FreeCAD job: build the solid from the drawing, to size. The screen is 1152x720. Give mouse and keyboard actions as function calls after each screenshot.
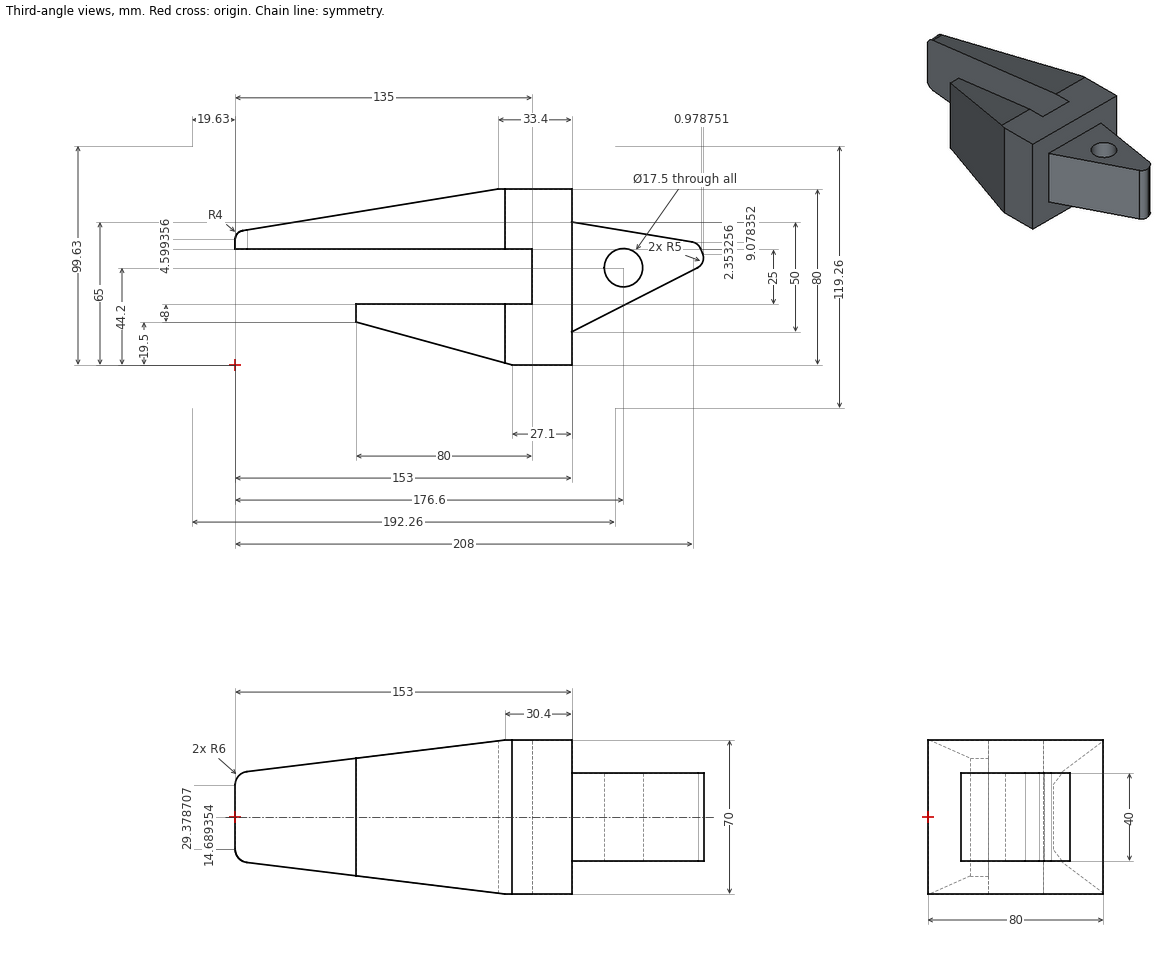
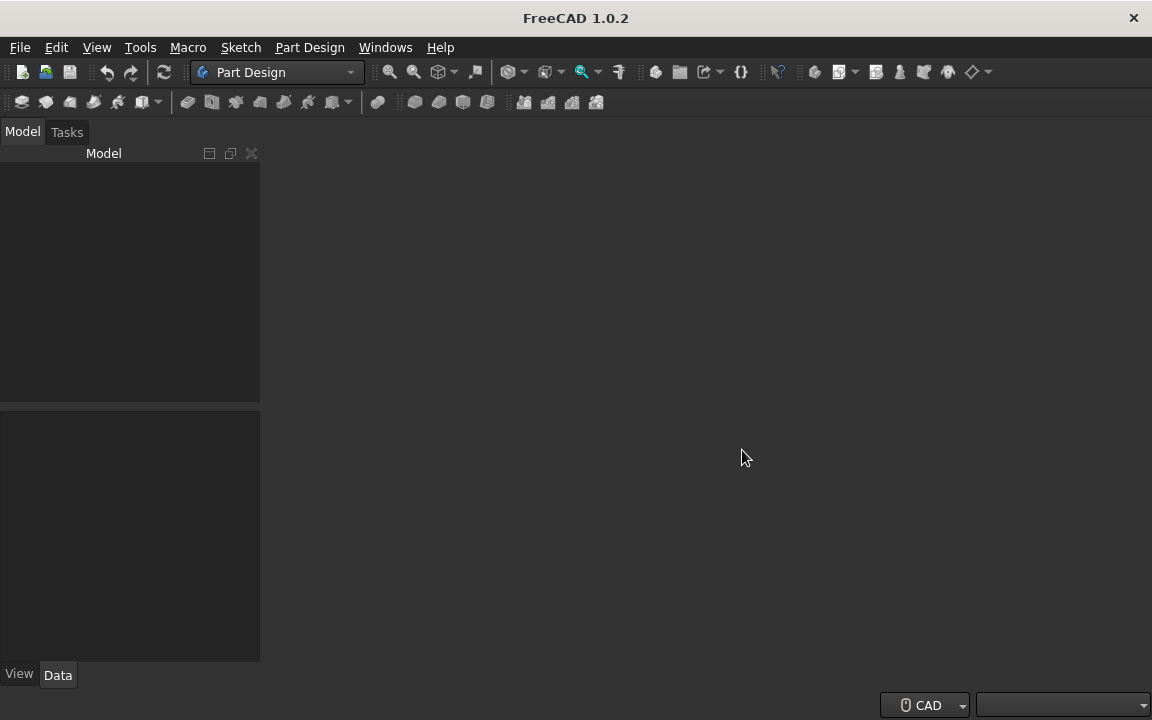
click(22, 72)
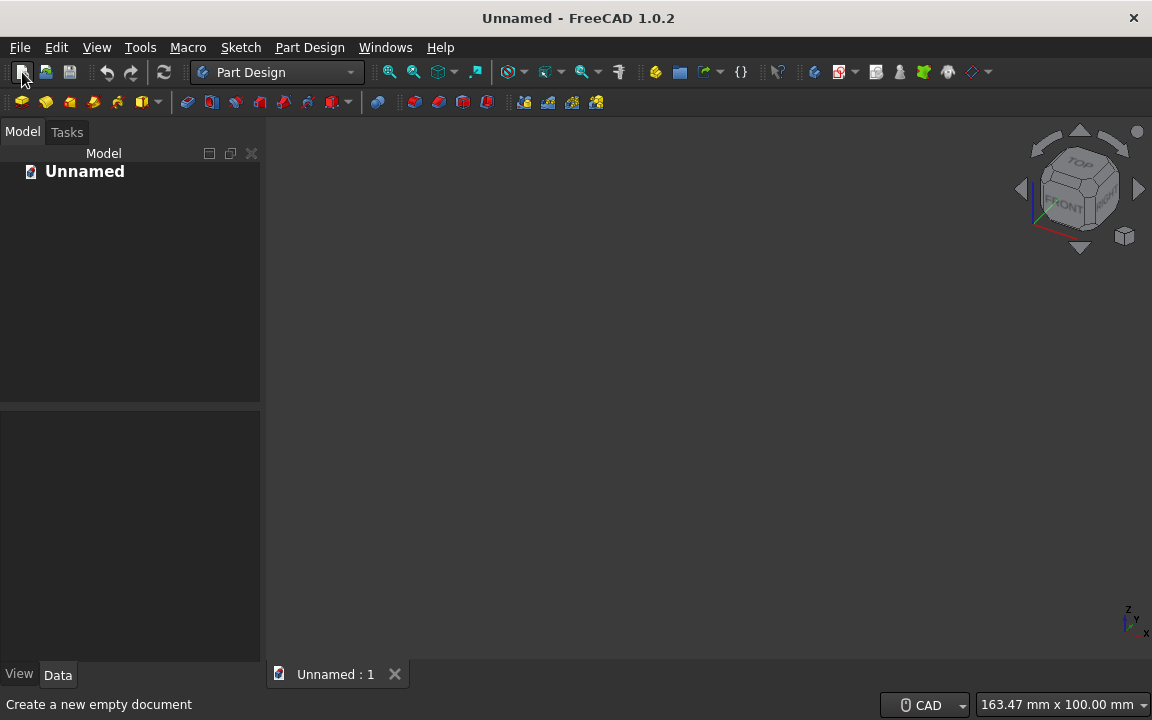
click(840, 72)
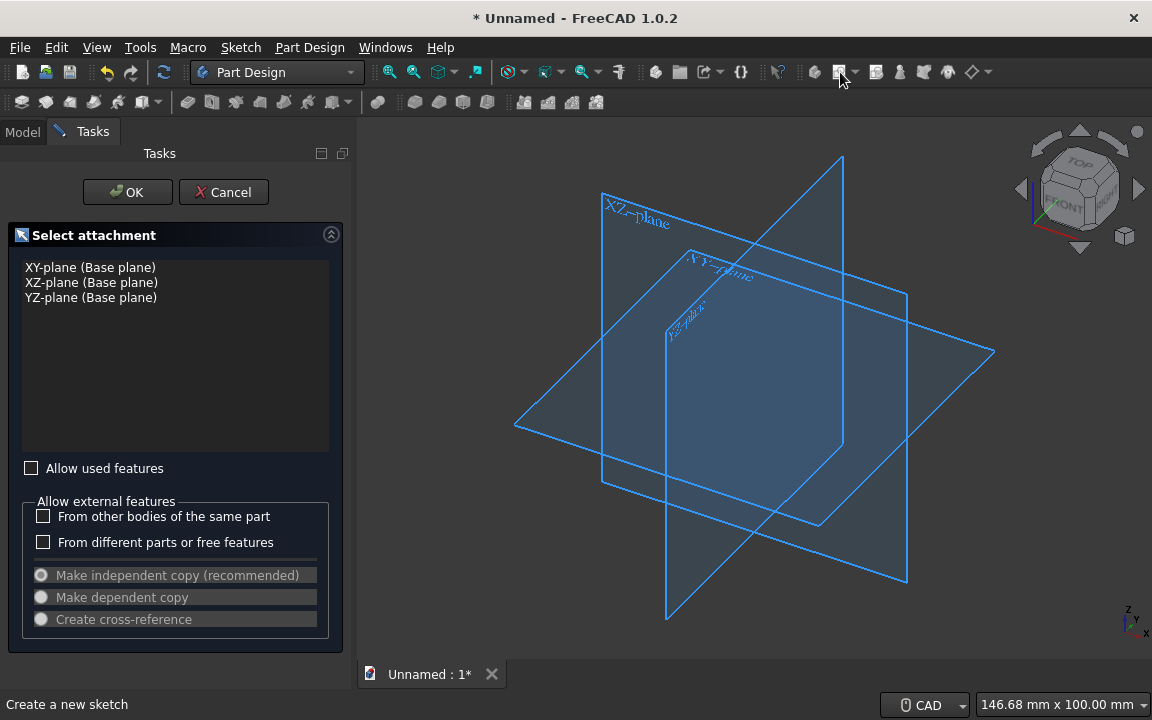
click(82, 282)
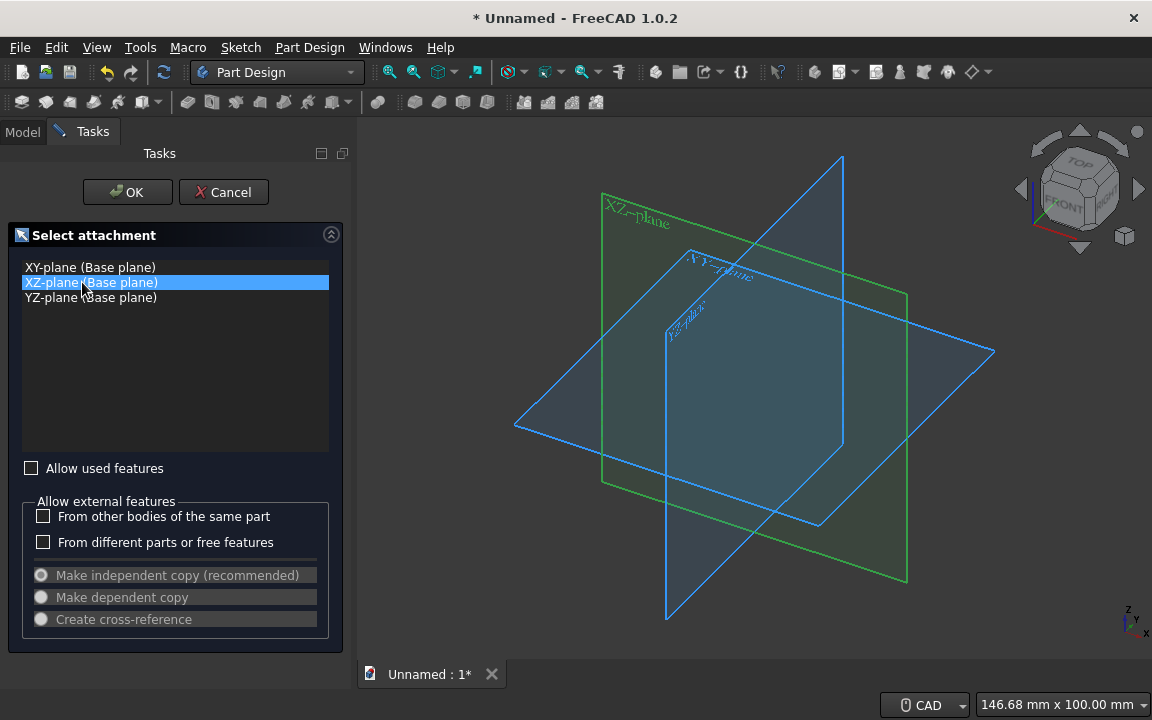
click(128, 192)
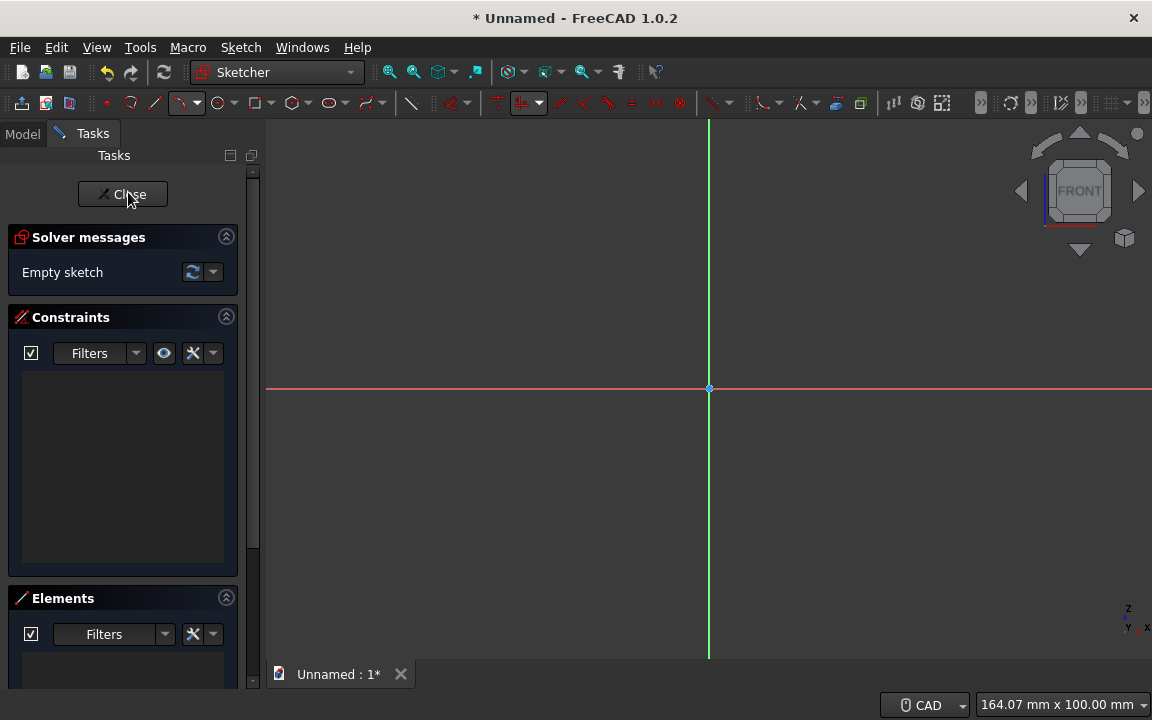
scroll(294, 389, down, 4)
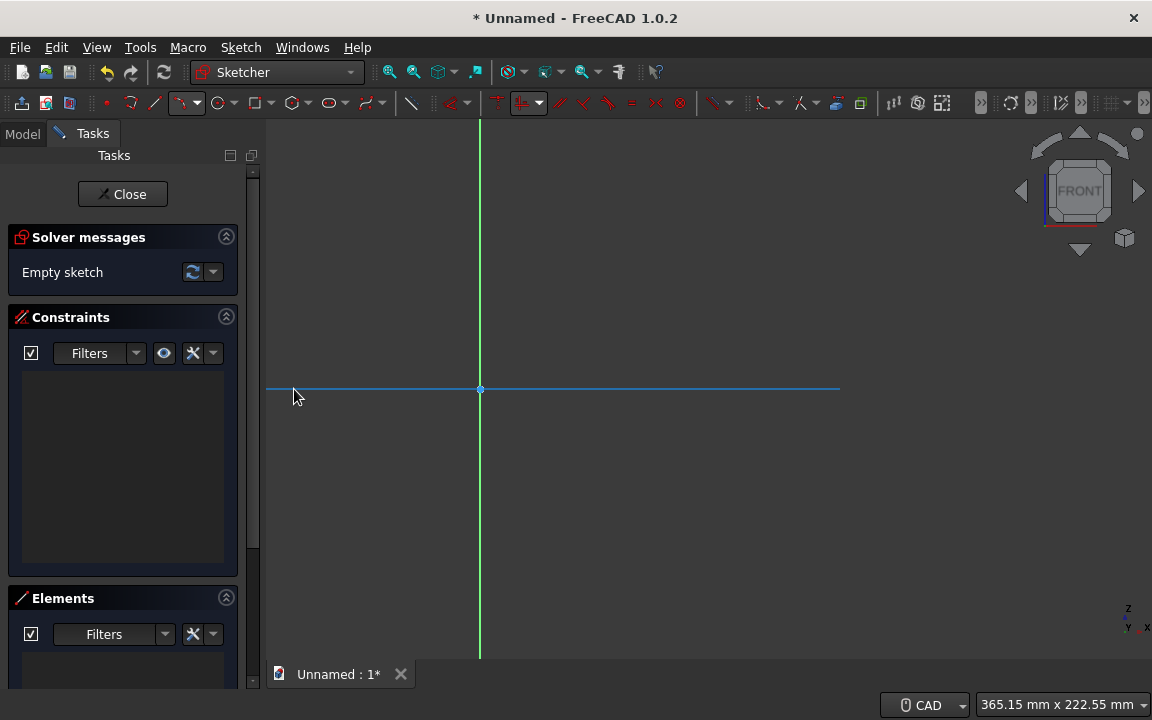
click(156, 104)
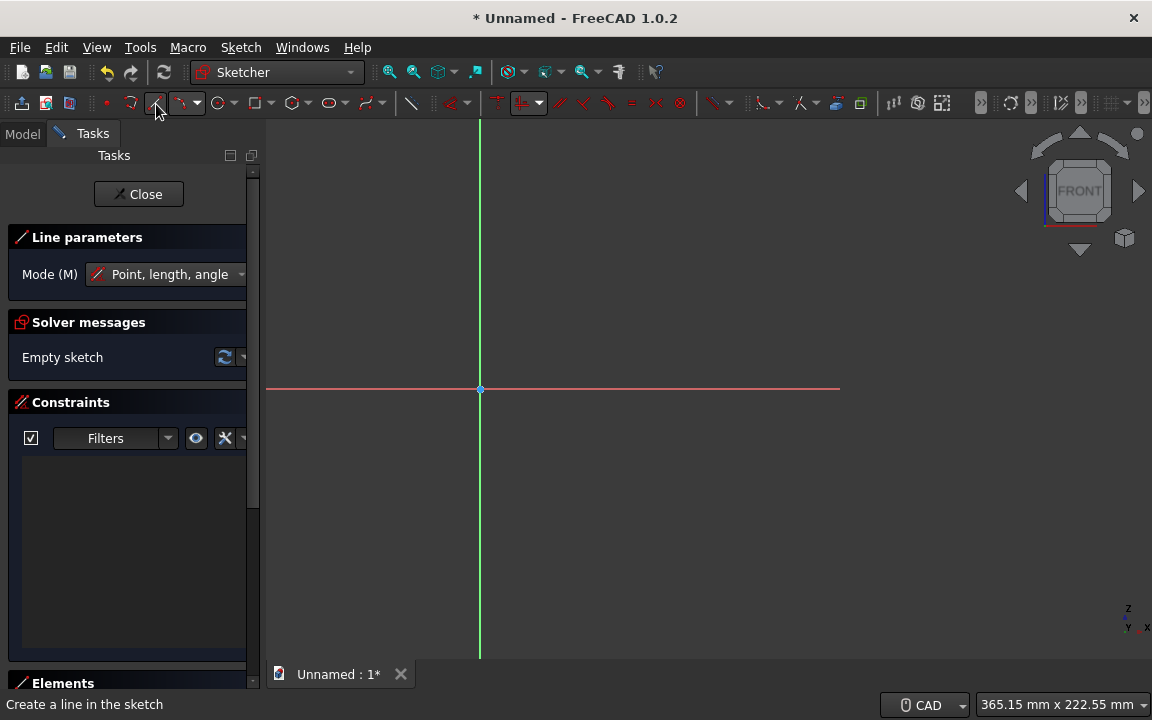
click(480, 425)
click(489, 354)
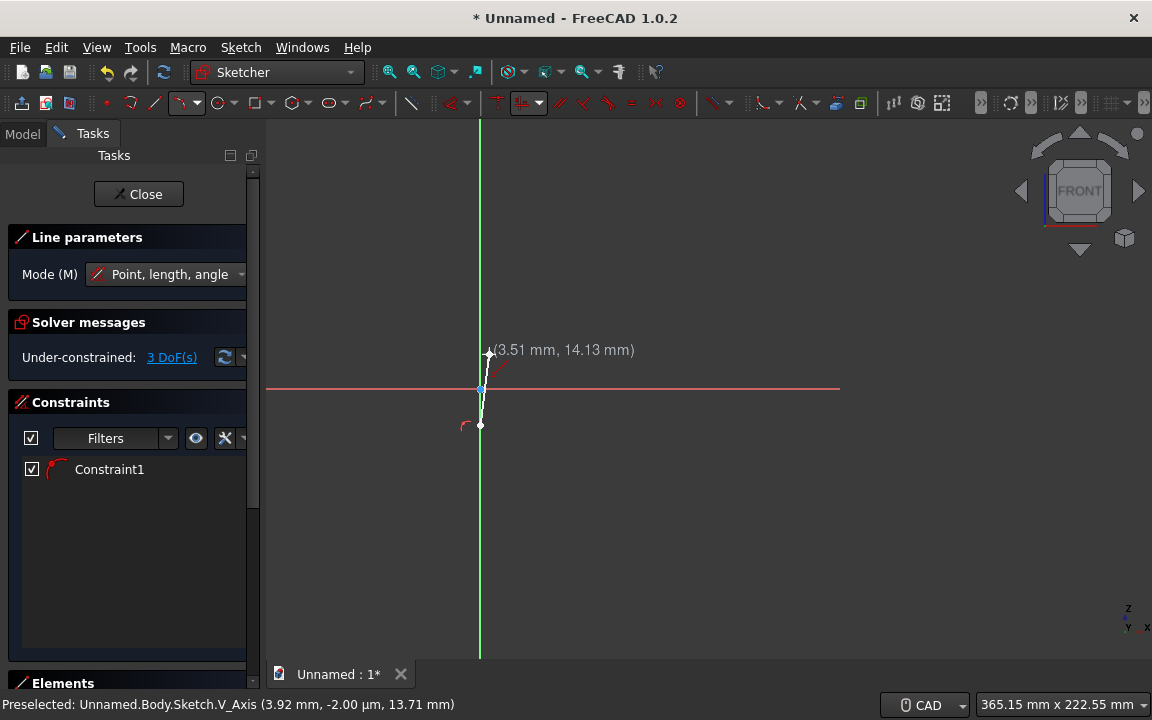
click(132, 104)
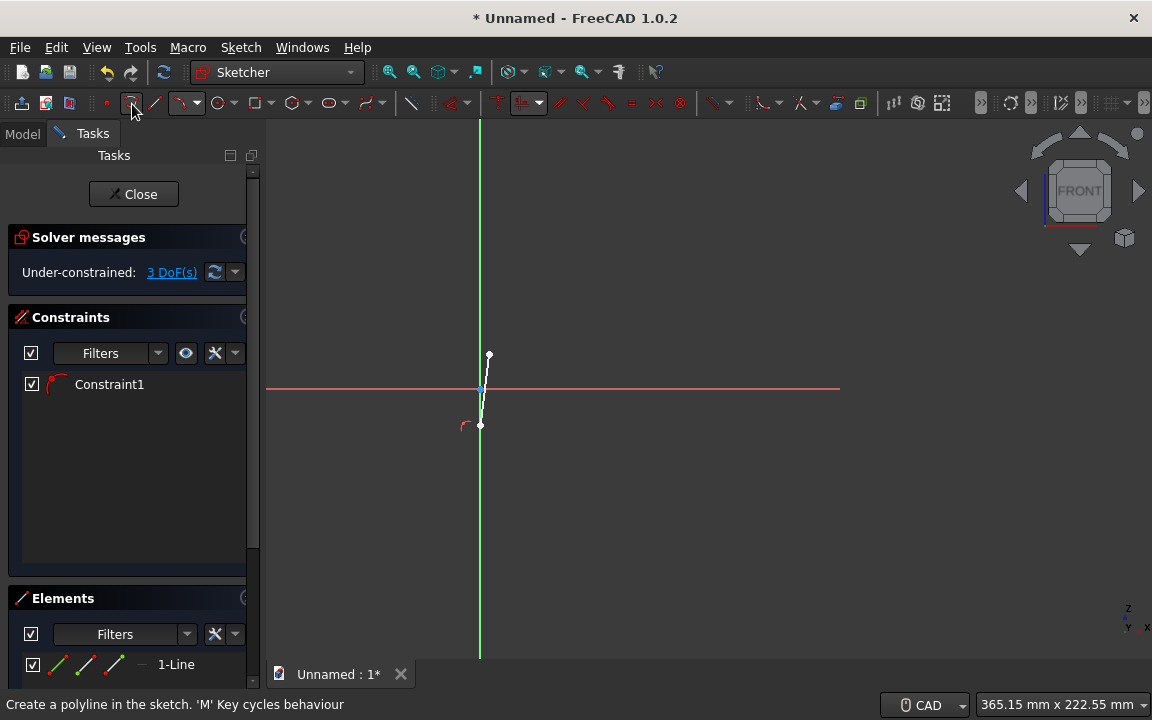
scroll(493, 339, up, 2)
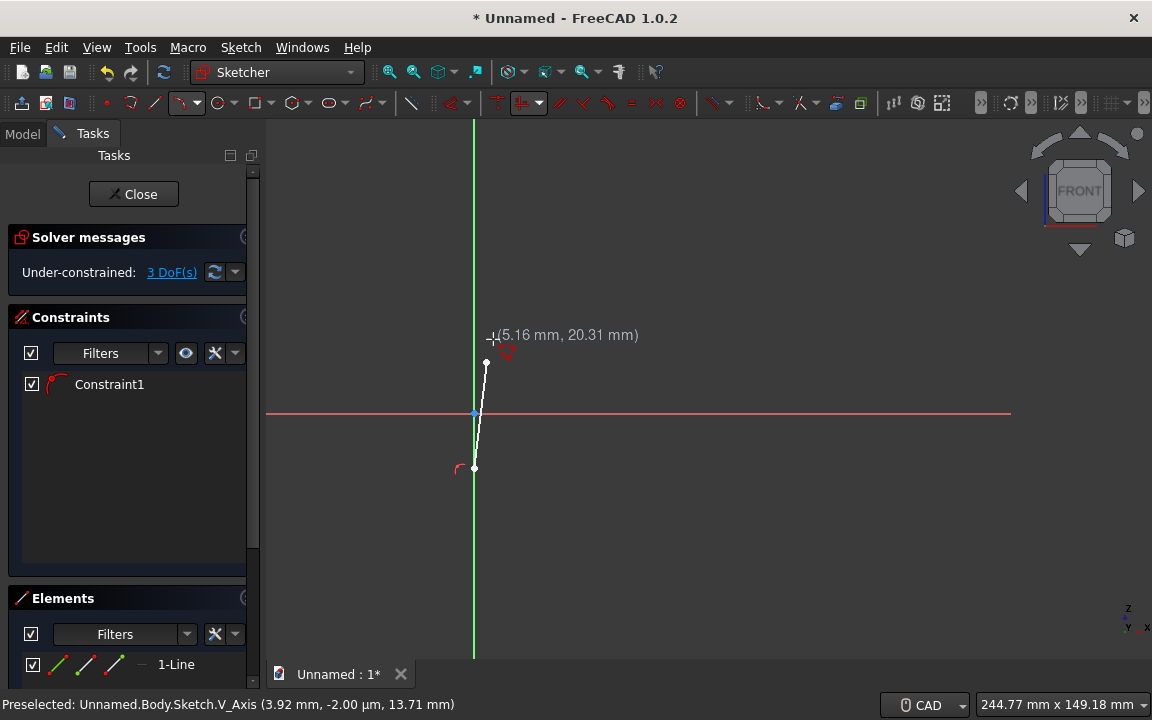
click(493, 339)
click(918, 287)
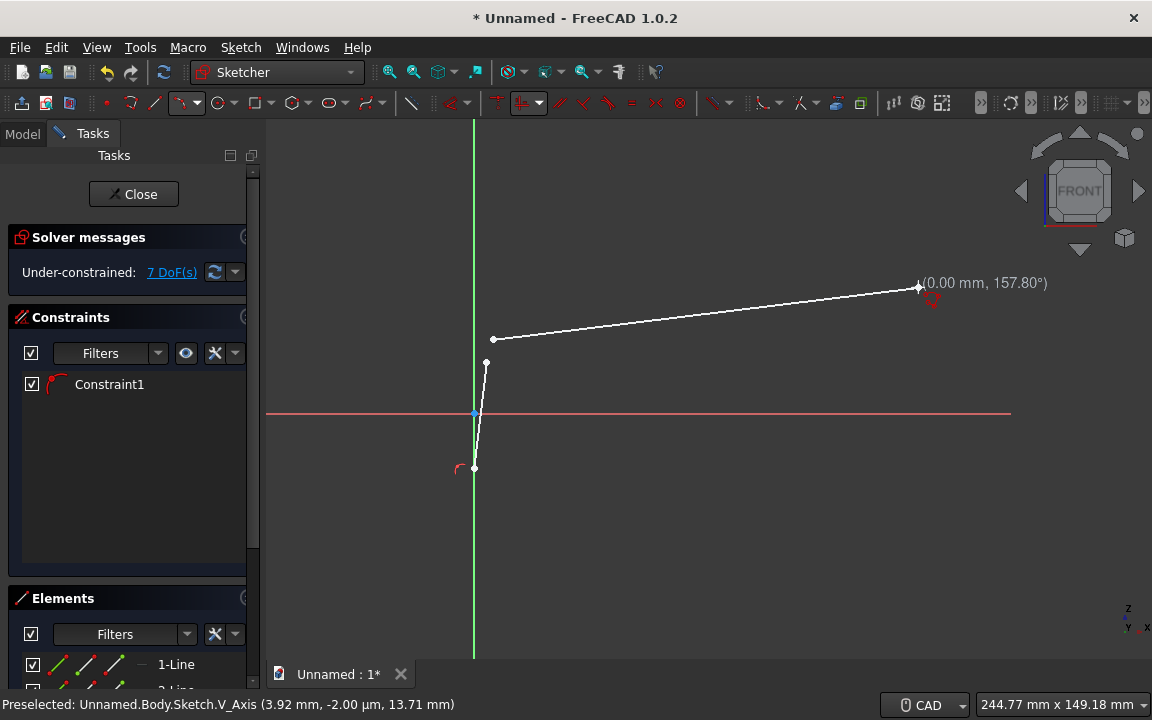
scroll(294, 277, down, 1)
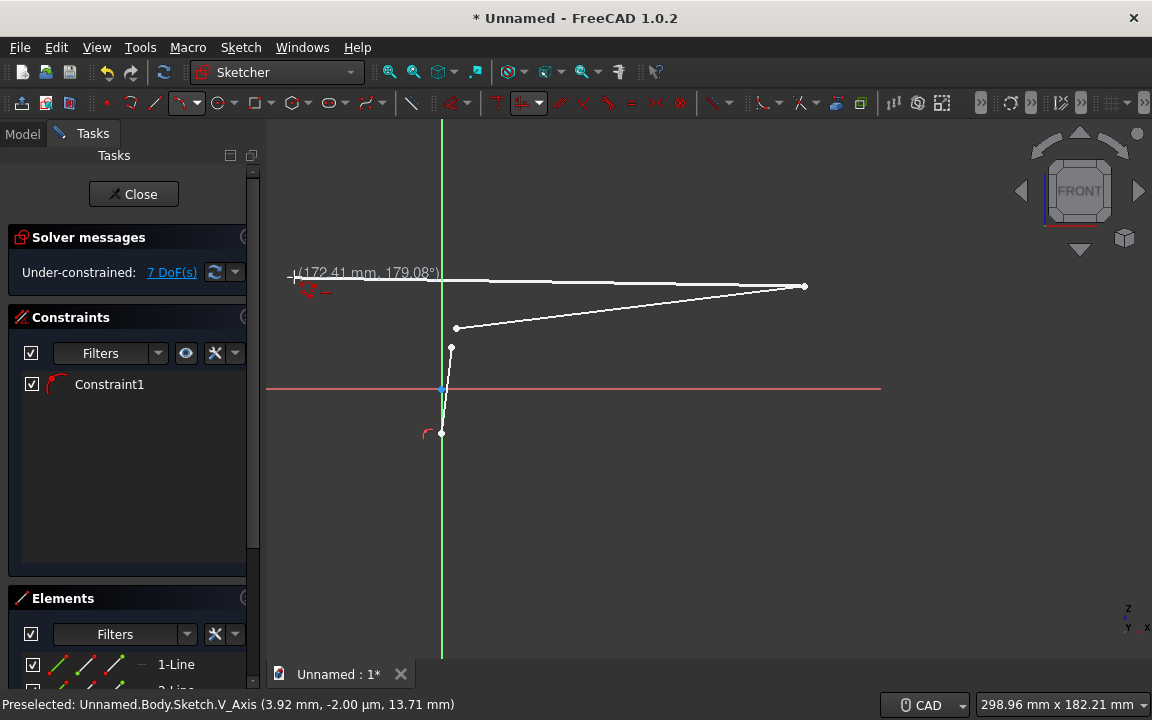
click(895, 285)
click(895, 493)
click(805, 493)
click(457, 450)
right_click(457, 450)